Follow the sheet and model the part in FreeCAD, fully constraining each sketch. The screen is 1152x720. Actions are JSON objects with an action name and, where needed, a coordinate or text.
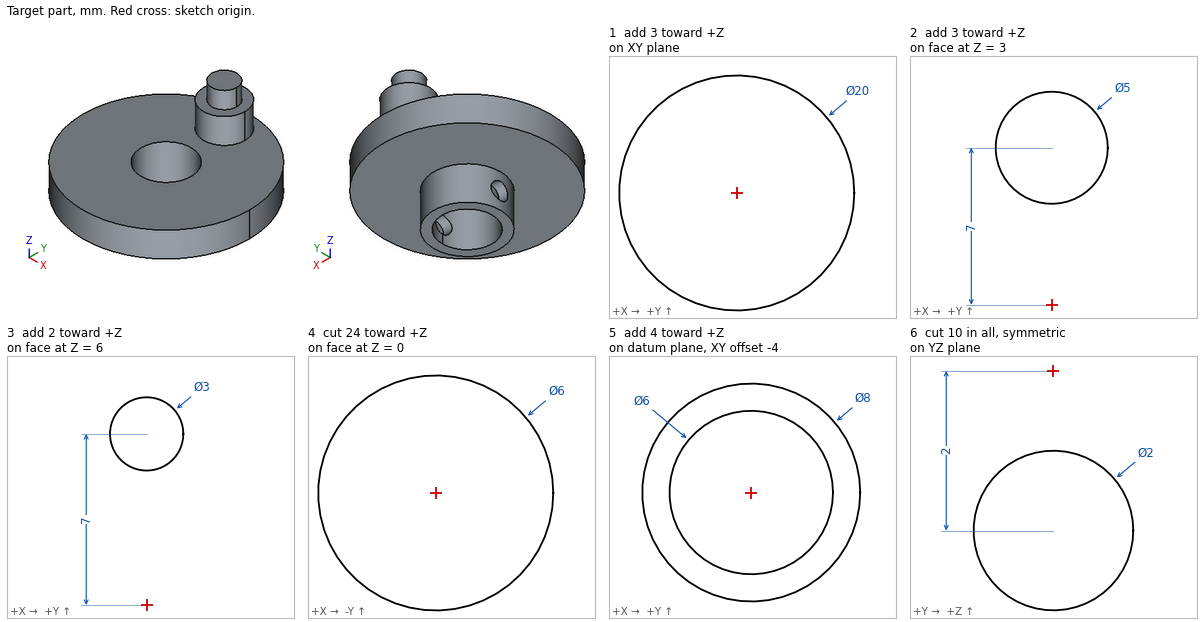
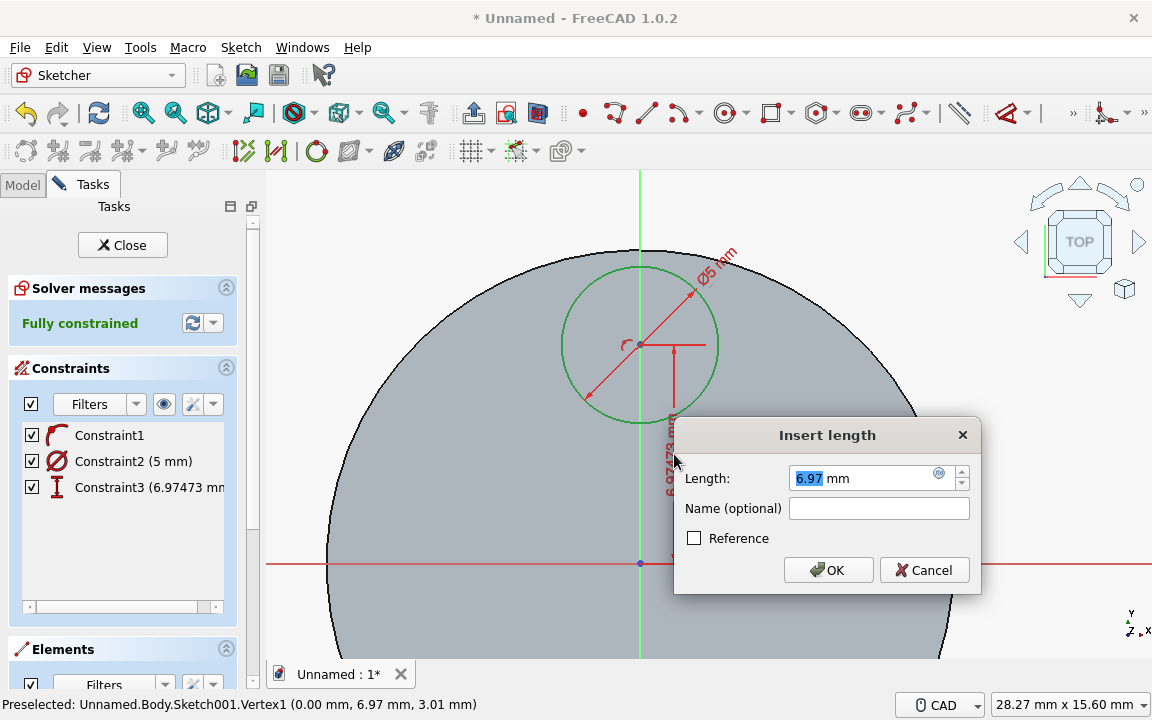
{"action": "type", "text": "7"}
{"action": "key", "text": "Return"}
{"action": "key", "text": "Escape"}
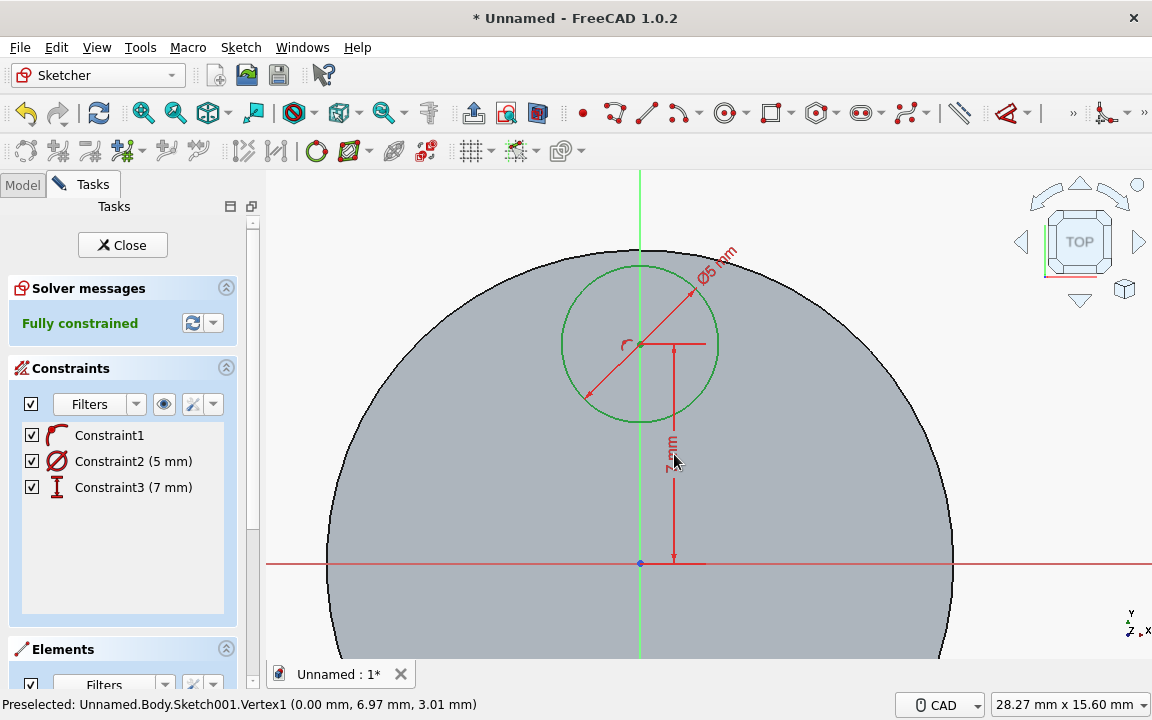
{"action": "left_click", "coordinate": [123, 245]}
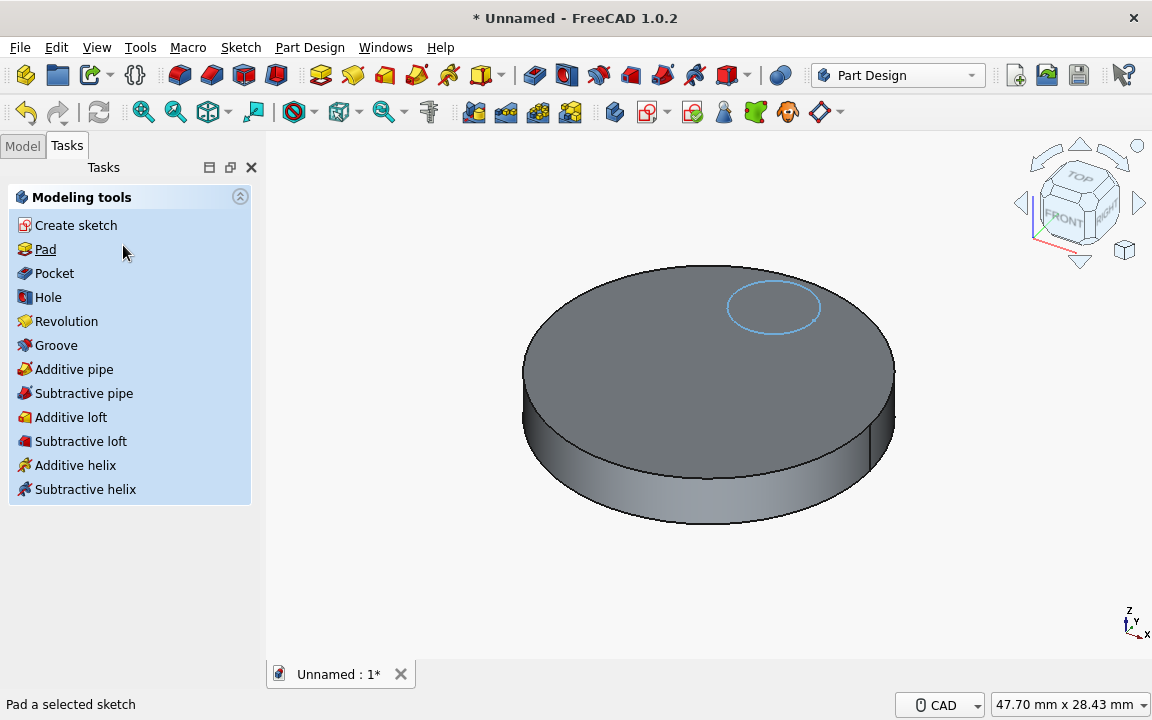
{"action": "left_click", "coordinate": [322, 76]}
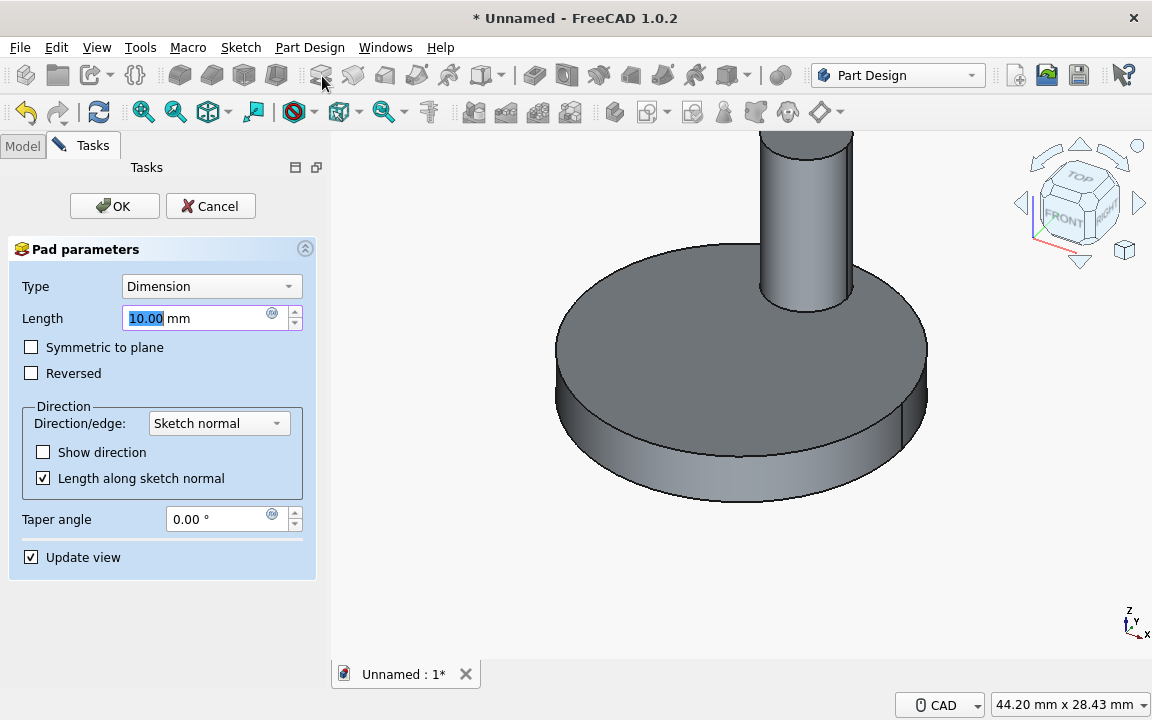
{"action": "type", "text": "3"}
{"action": "key", "text": "Tab"}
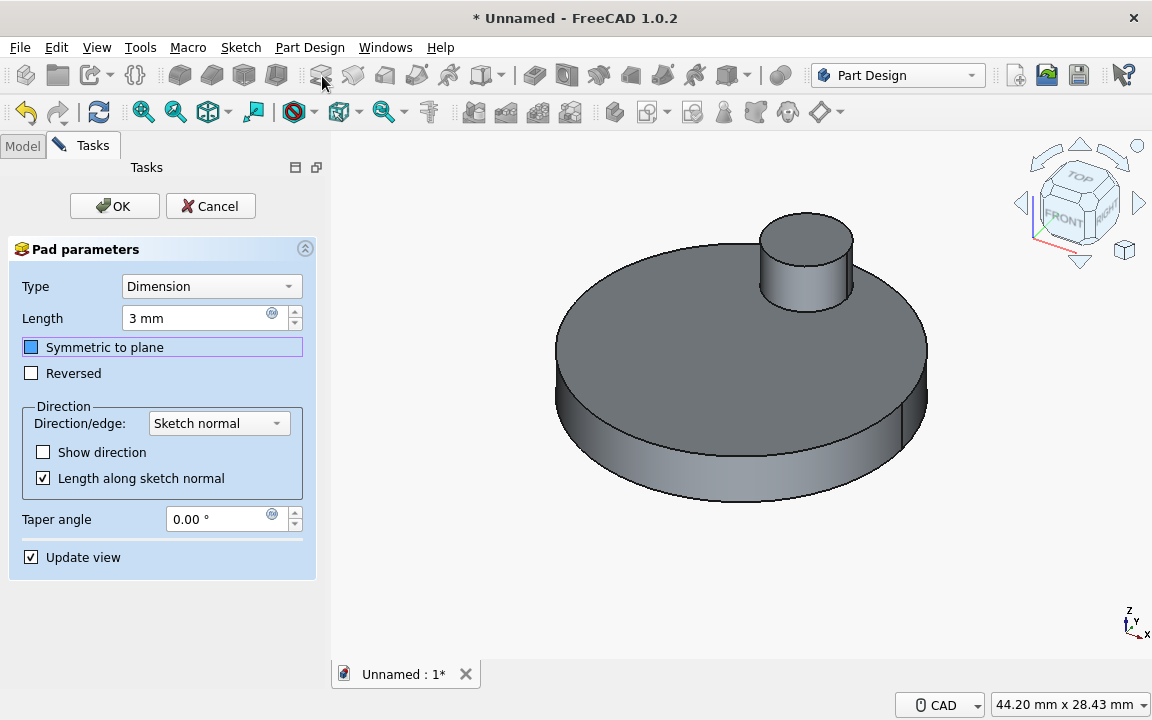
{"action": "left_click", "coordinate": [115, 206]}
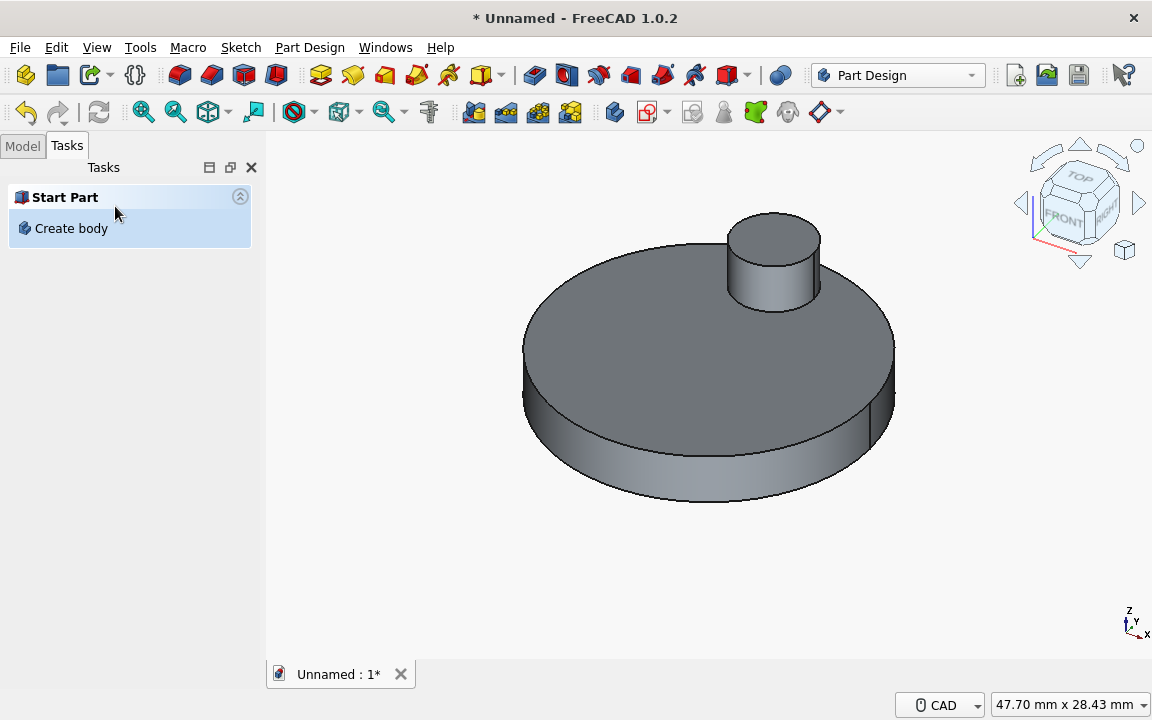
{"action": "left_click", "coordinate": [774, 239]}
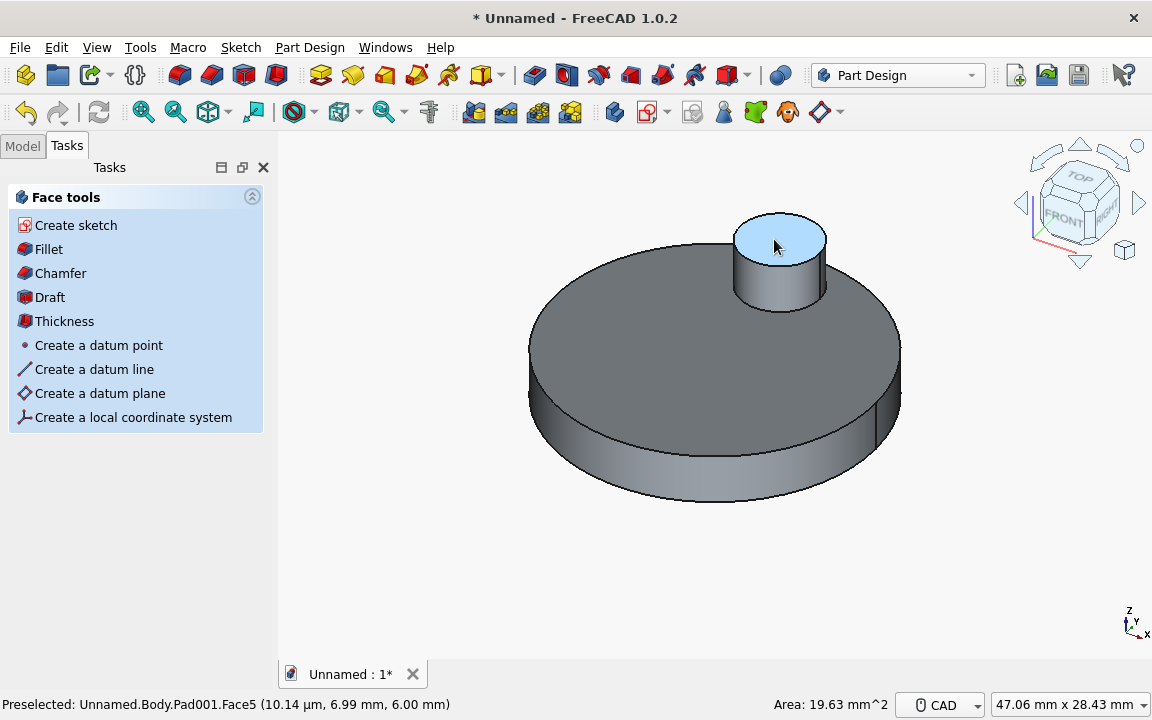
{"action": "left_click", "coordinate": [648, 112]}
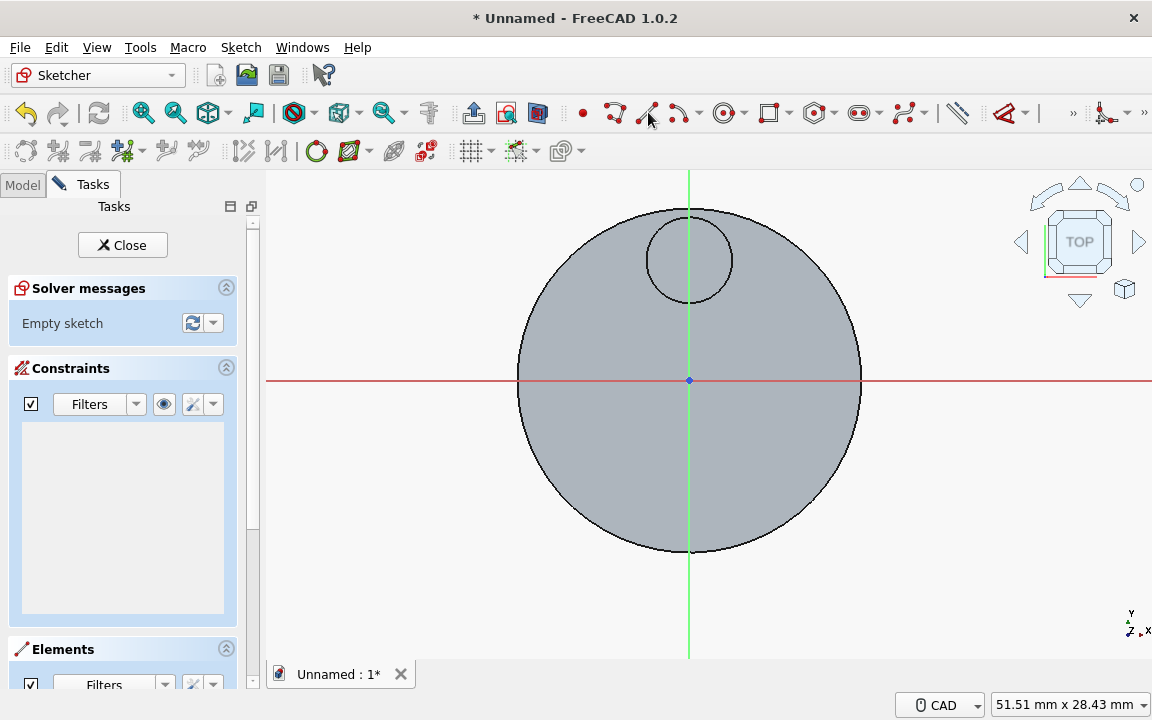
{"action": "scroll", "coordinate": [699, 230], "scroll_direction": "up", "scroll_amount": 9}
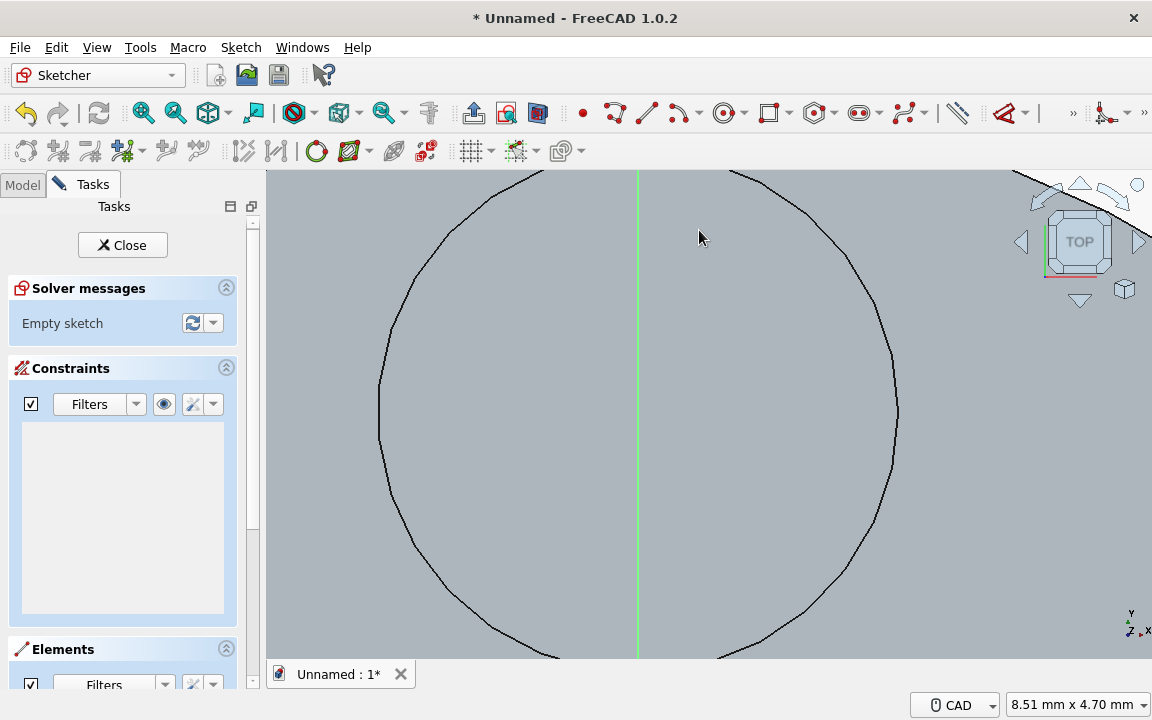
{"action": "left_click", "coordinate": [724, 114]}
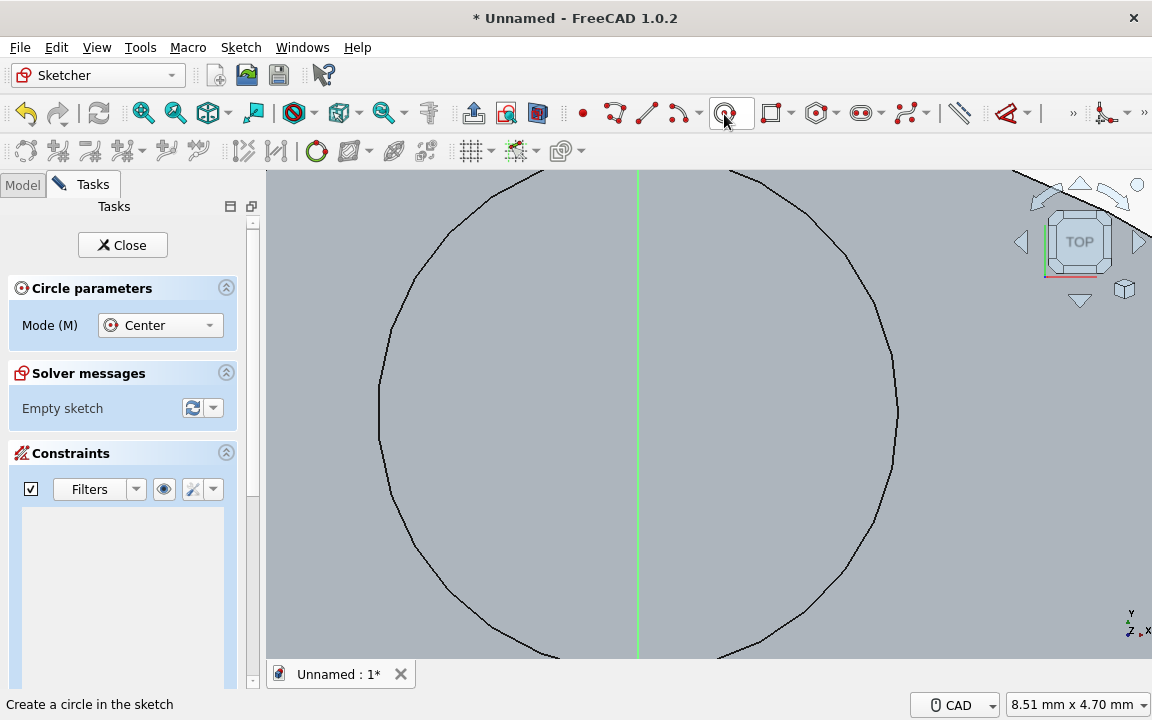
{"action": "left_click", "coordinate": [638, 412]}
{"action": "left_click", "coordinate": [748, 302]}
{"action": "key", "text": "Escape"}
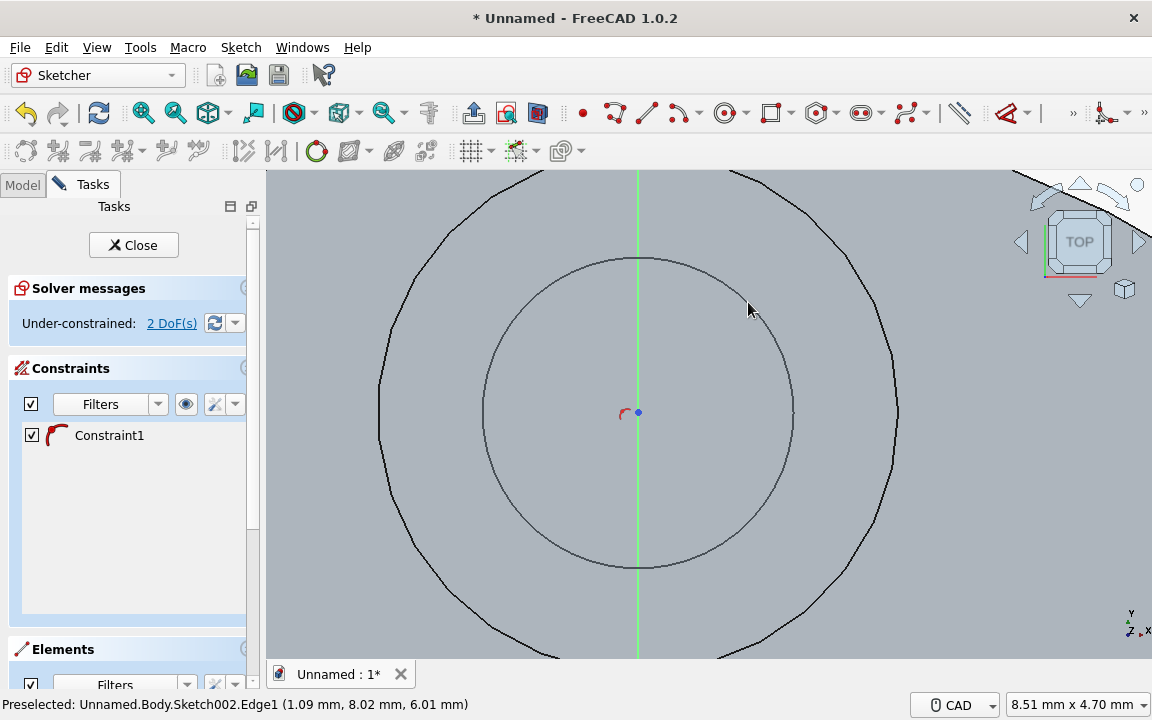
{"action": "key", "text": "d"}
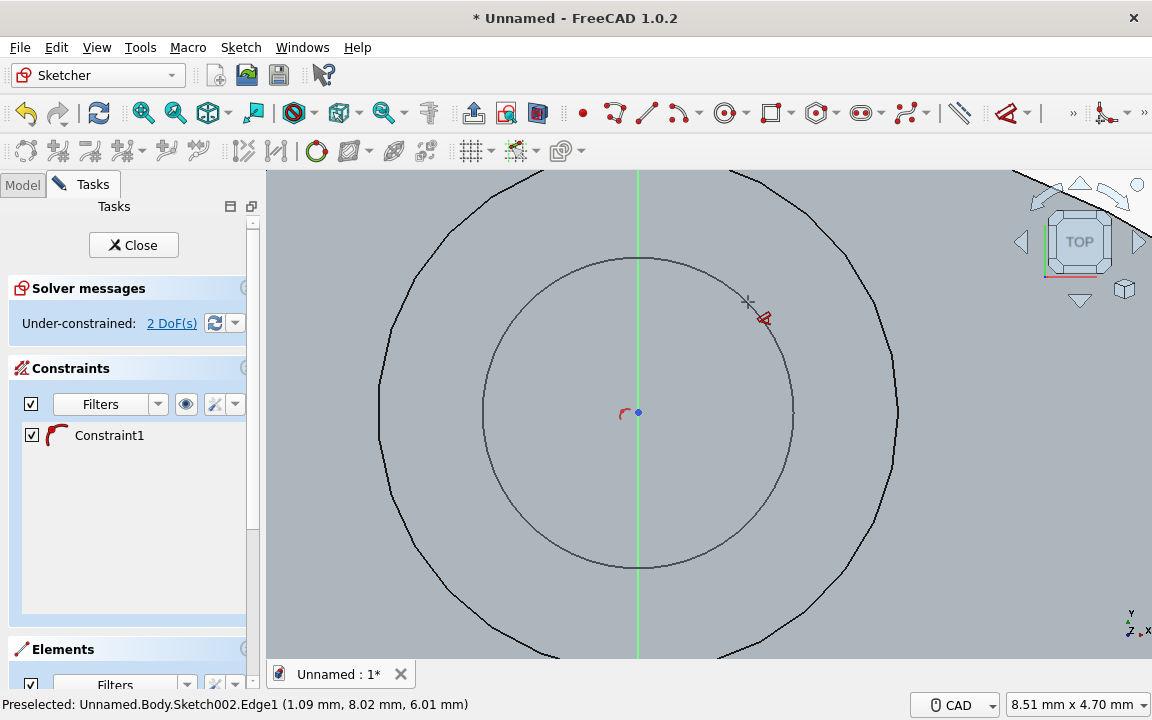
{"action": "left_click", "coordinate": [748, 303]}
{"action": "left_click", "coordinate": [771, 280]}